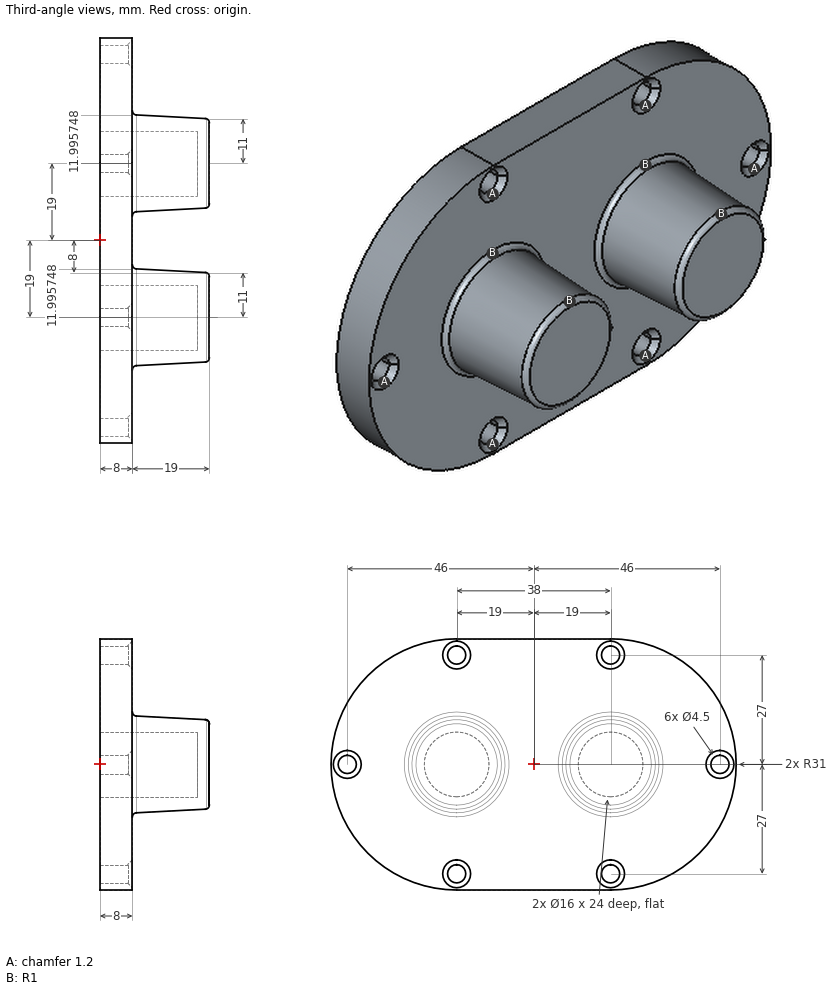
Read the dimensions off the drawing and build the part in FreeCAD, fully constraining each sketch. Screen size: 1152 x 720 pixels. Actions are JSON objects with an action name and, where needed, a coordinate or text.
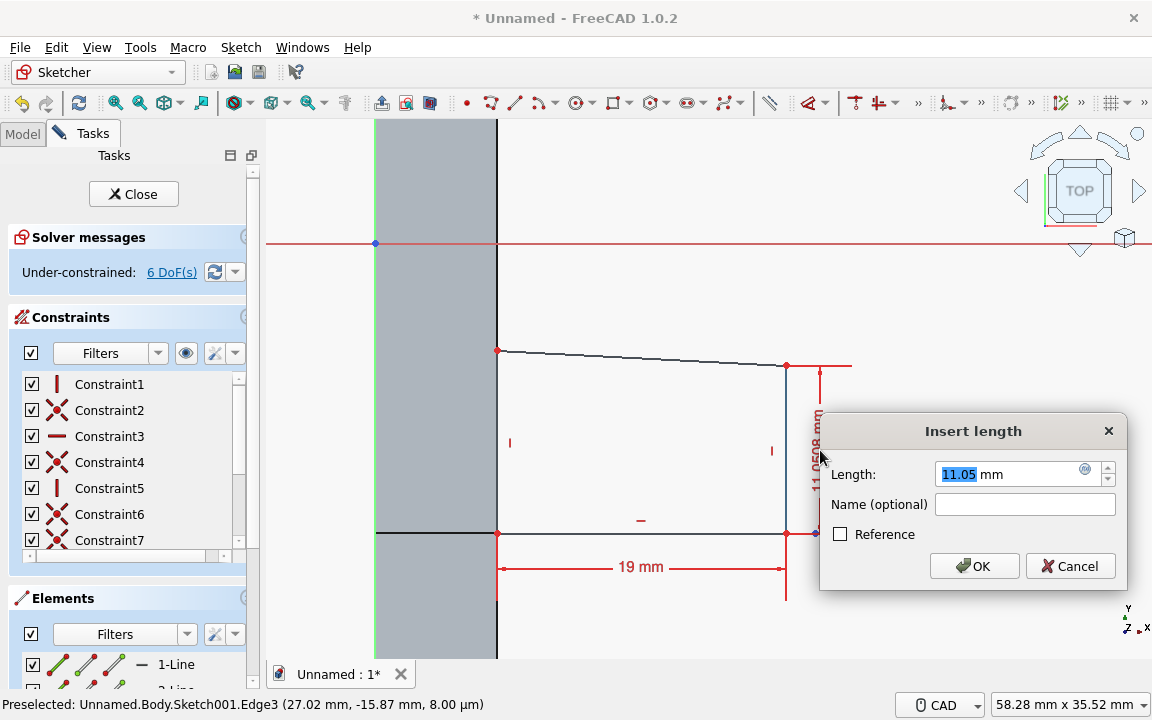
{"action": "type", "text": "11"}
{"action": "key", "text": "Return"}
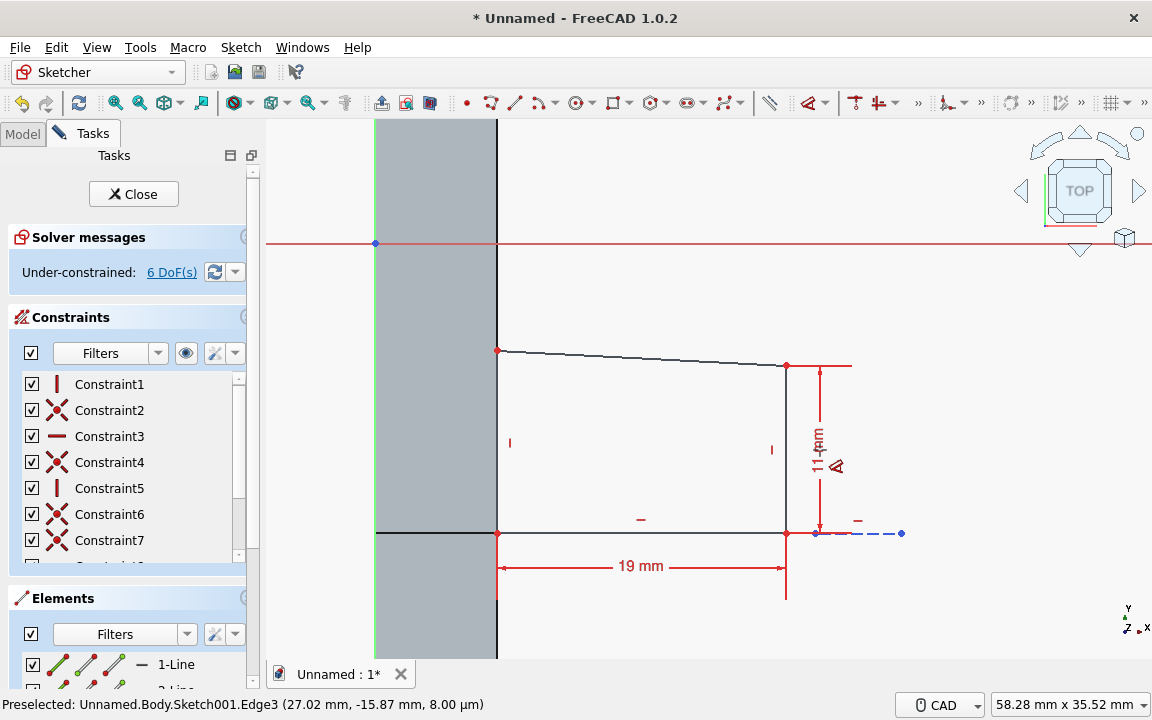
{"action": "left_click", "coordinate": [497, 351]}
{"action": "left_click", "coordinate": [436, 210]}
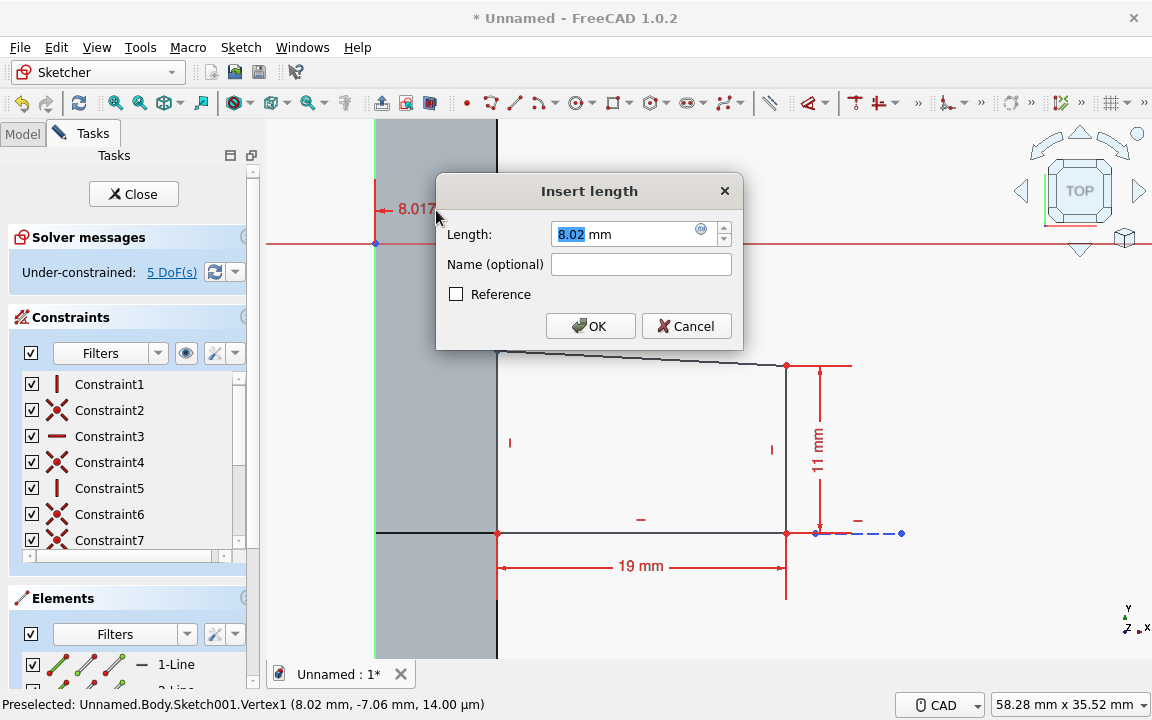
{"action": "type", "text": "8"}
{"action": "key", "text": "Return"}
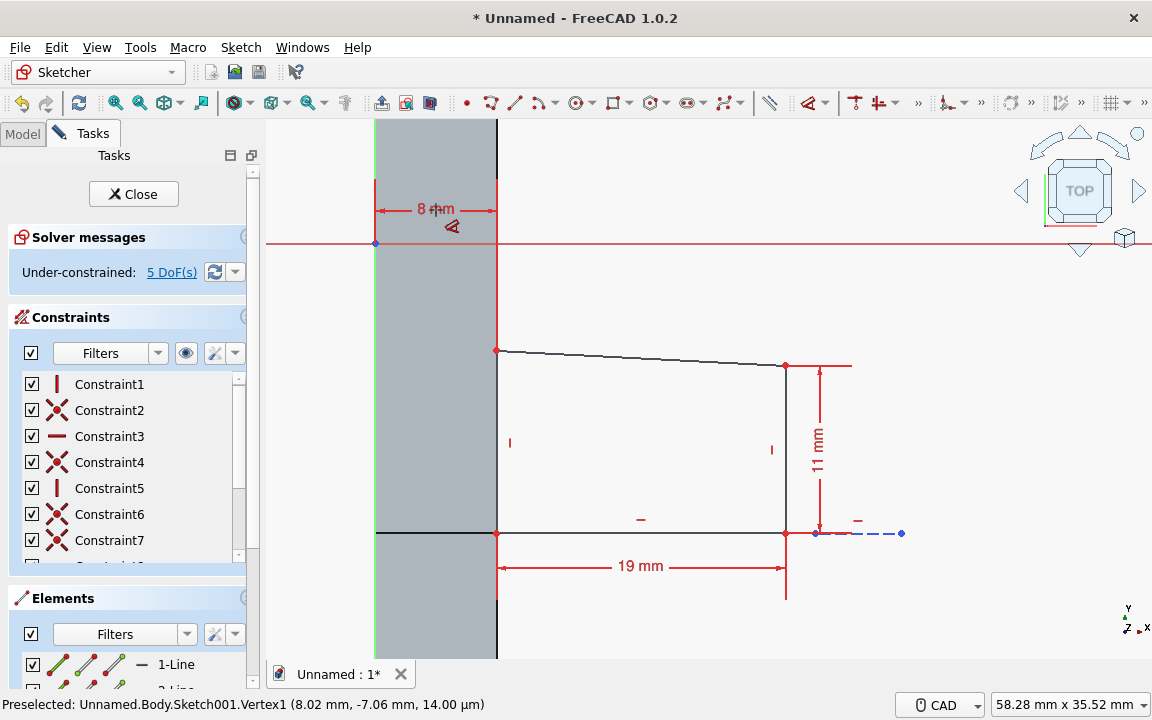
{"action": "left_click", "coordinate": [786, 366]}
{"action": "left_click", "coordinate": [341, 305]}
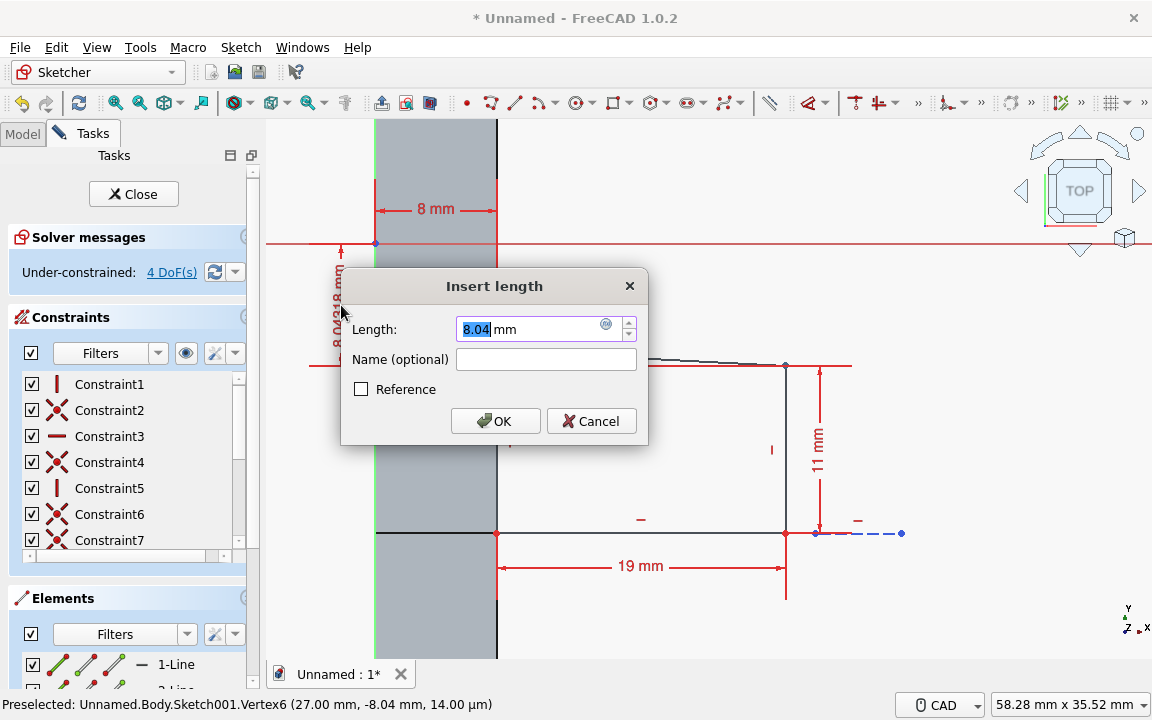
{"action": "type", "text": "8"}
{"action": "key", "text": "Return"}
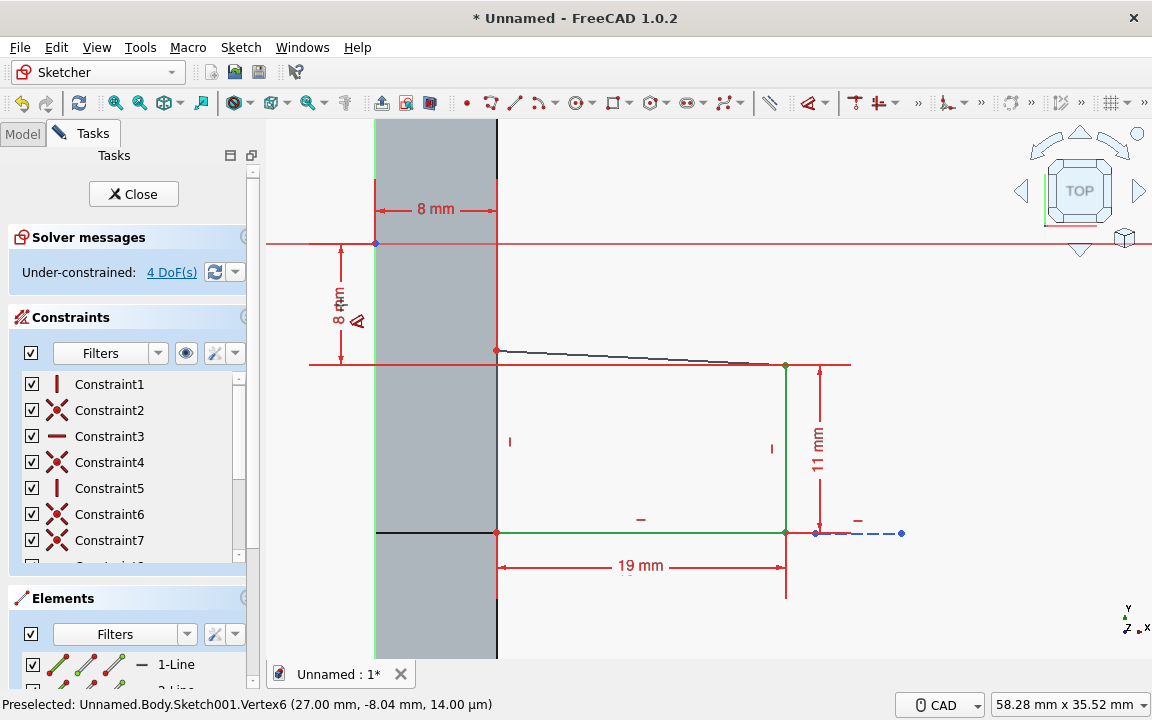
{"action": "left_click", "coordinate": [815, 534]}
{"action": "left_click", "coordinate": [341, 389]}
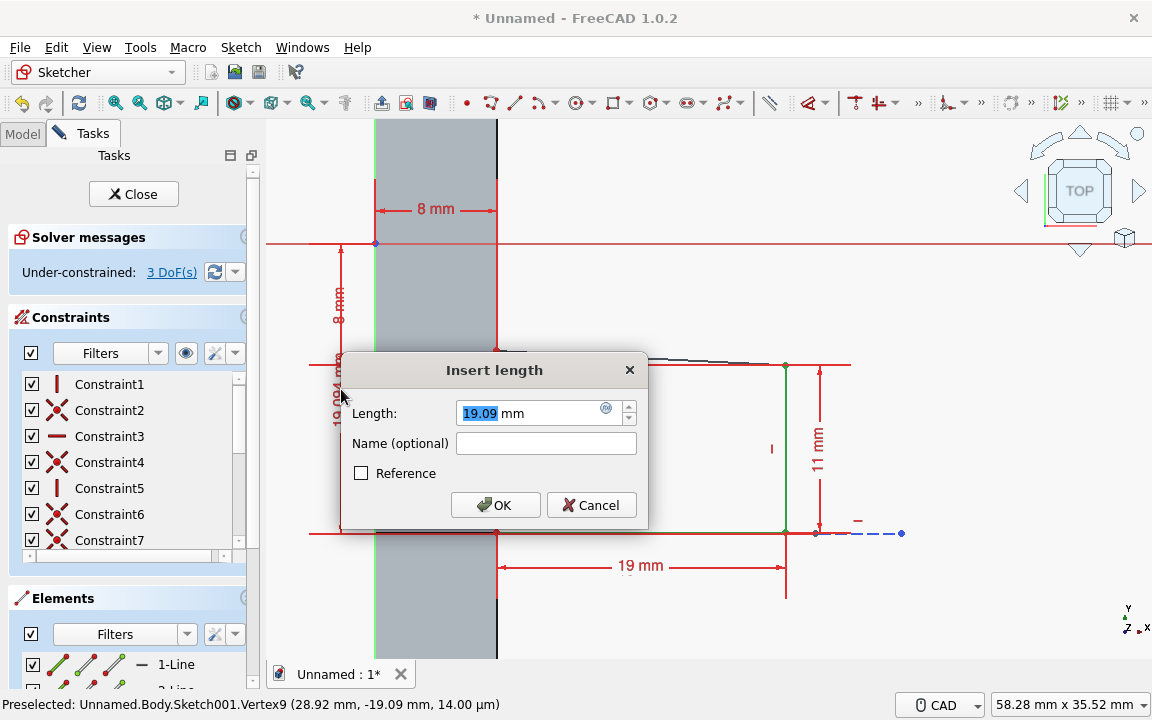
{"action": "type", "text": "19"}
{"action": "key", "text": "Return"}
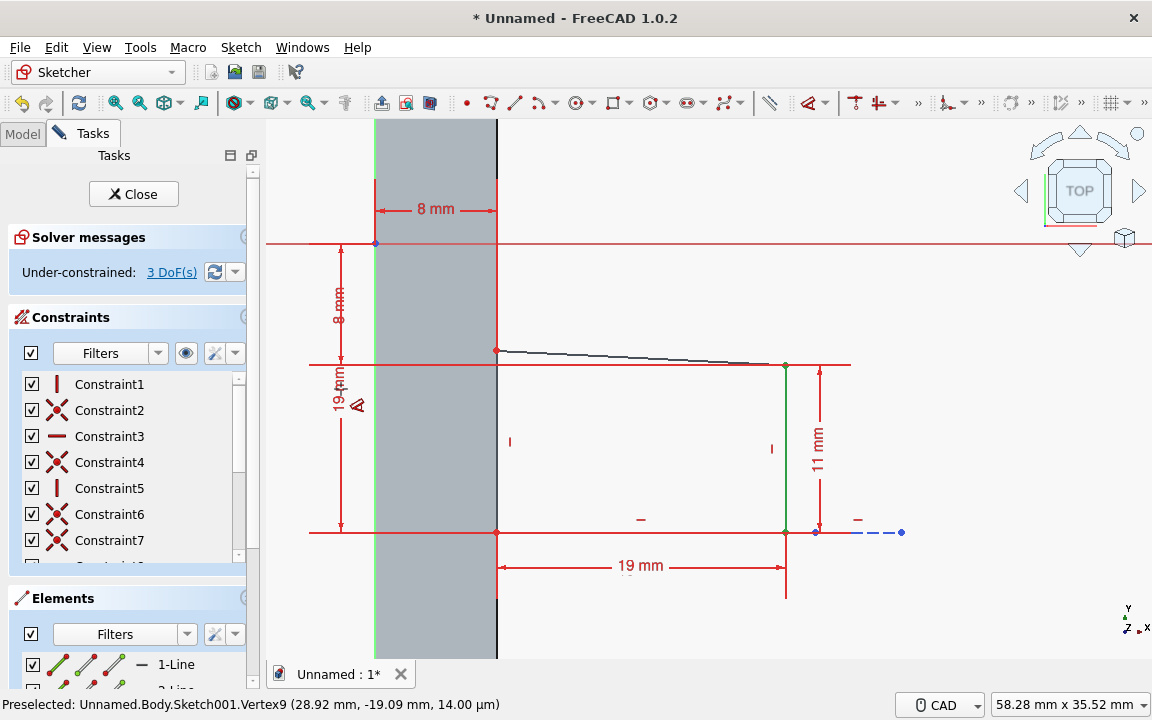
{"action": "left_click", "coordinate": [497, 405]}
{"action": "left_click", "coordinate": [463, 442]}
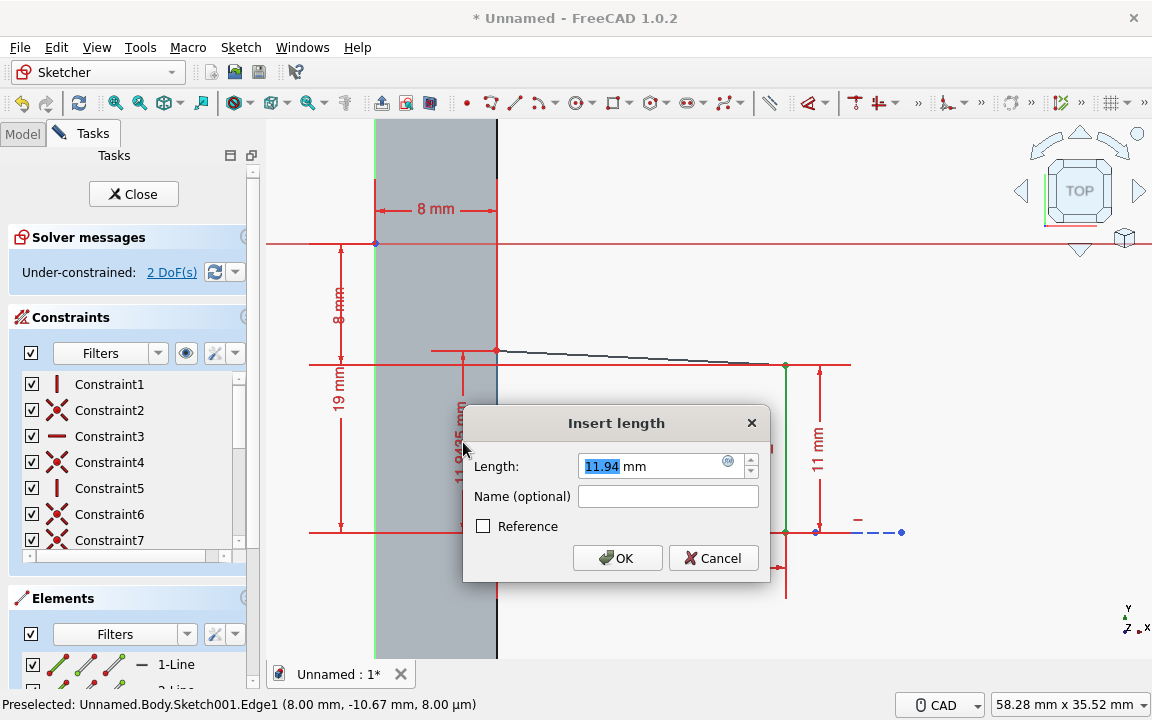
{"action": "type", "text": "11.995748"}
{"action": "key", "text": "Return"}
{"action": "key", "text": "Escape"}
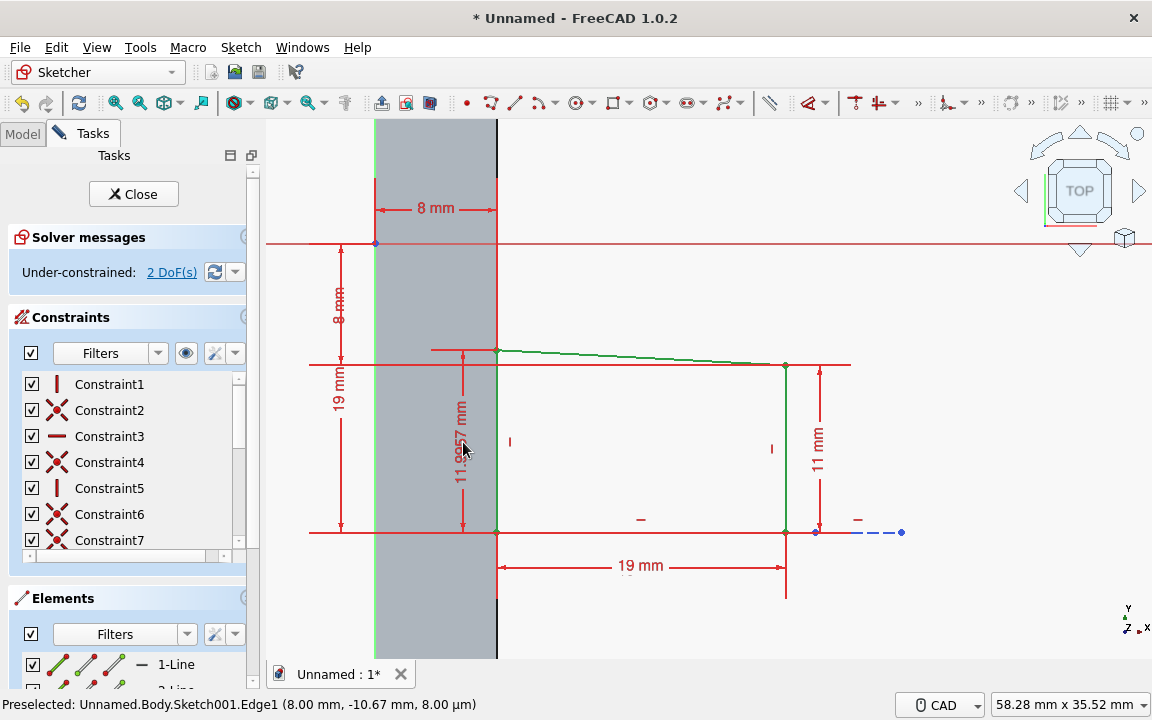
{"action": "left_click", "coordinate": [134, 194]}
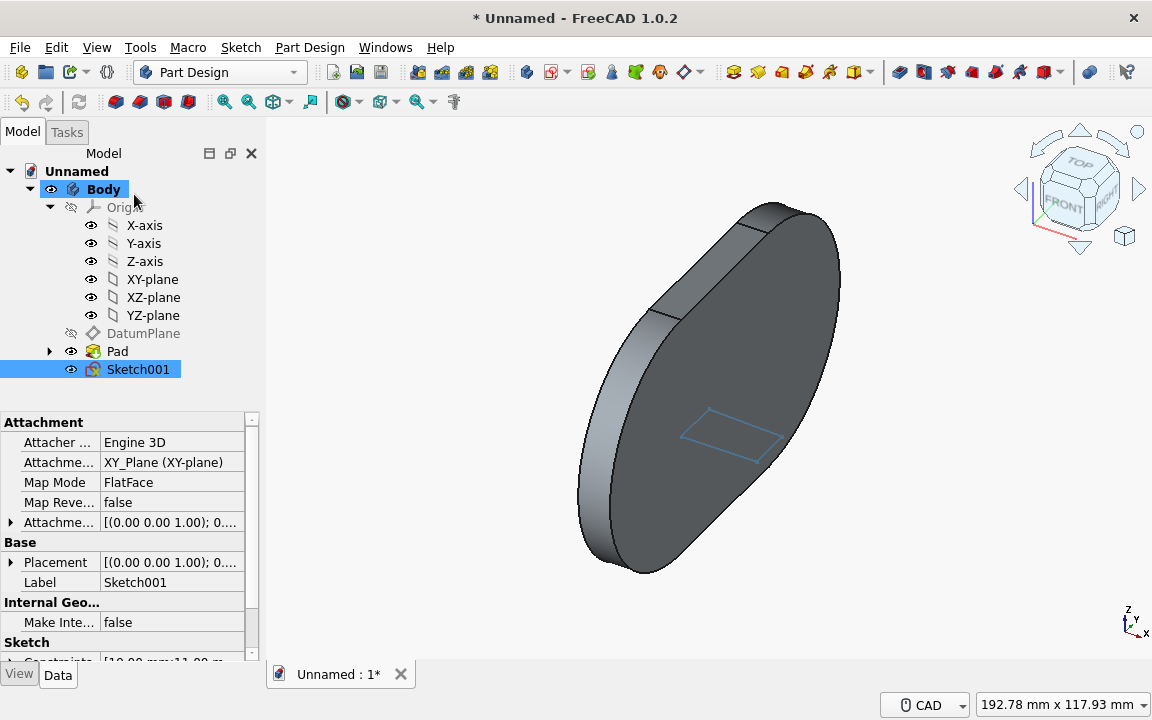
{"action": "left_click", "coordinate": [758, 72]}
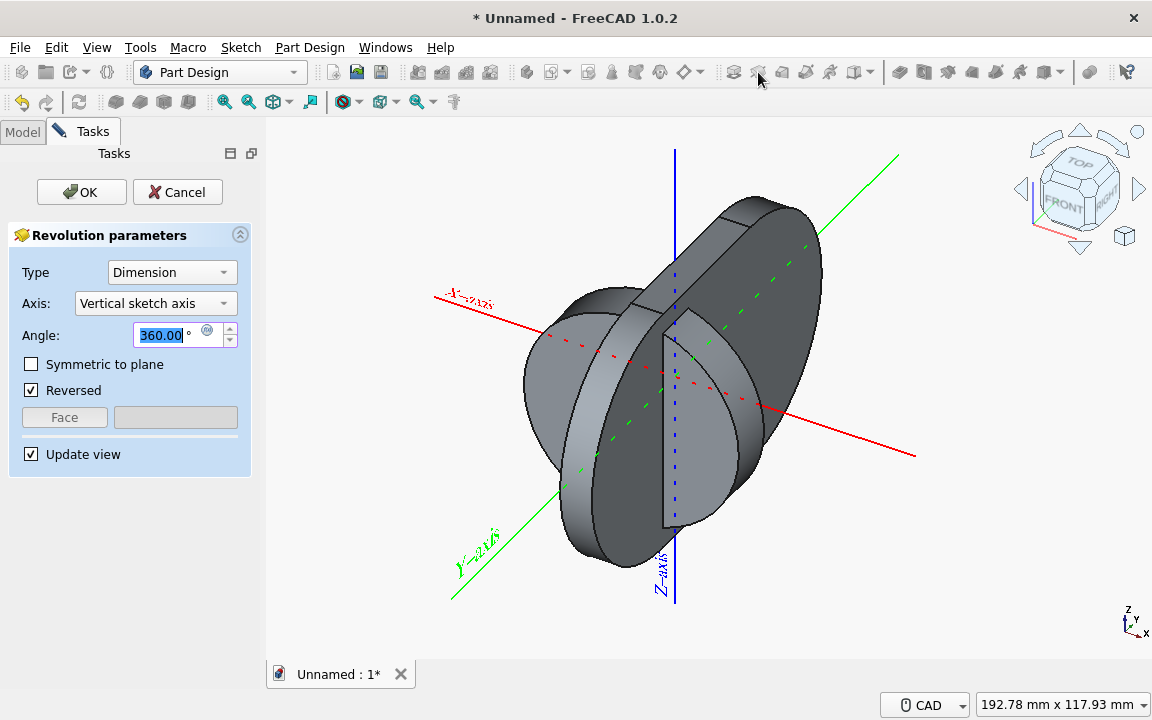
{"action": "left_click", "coordinate": [156, 304]}